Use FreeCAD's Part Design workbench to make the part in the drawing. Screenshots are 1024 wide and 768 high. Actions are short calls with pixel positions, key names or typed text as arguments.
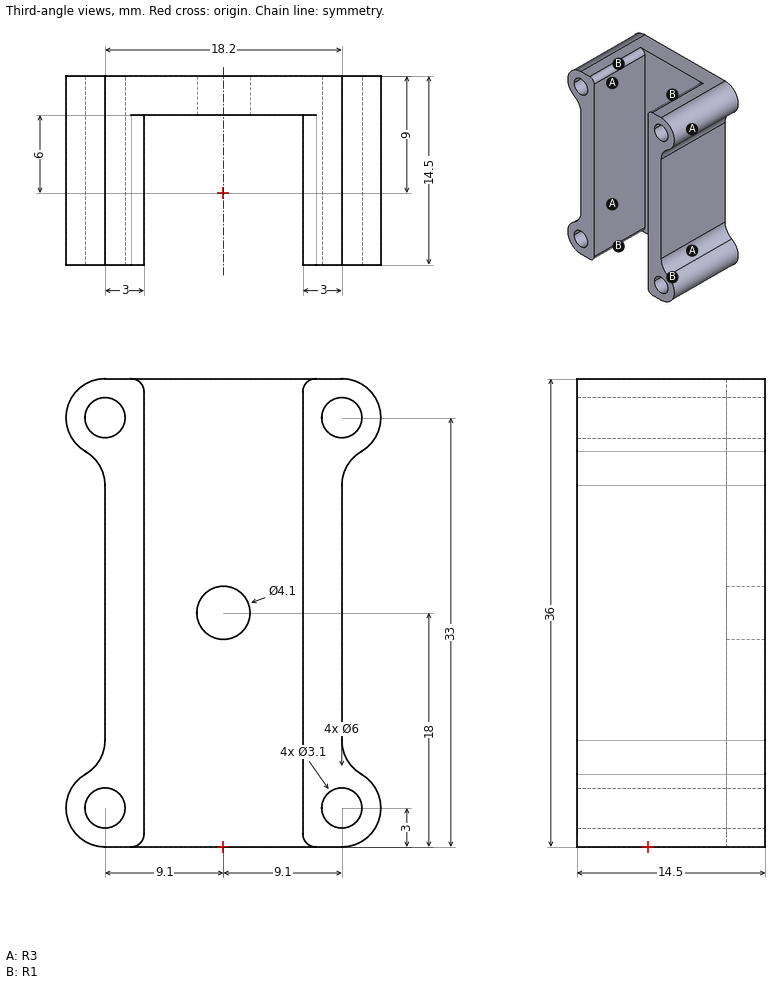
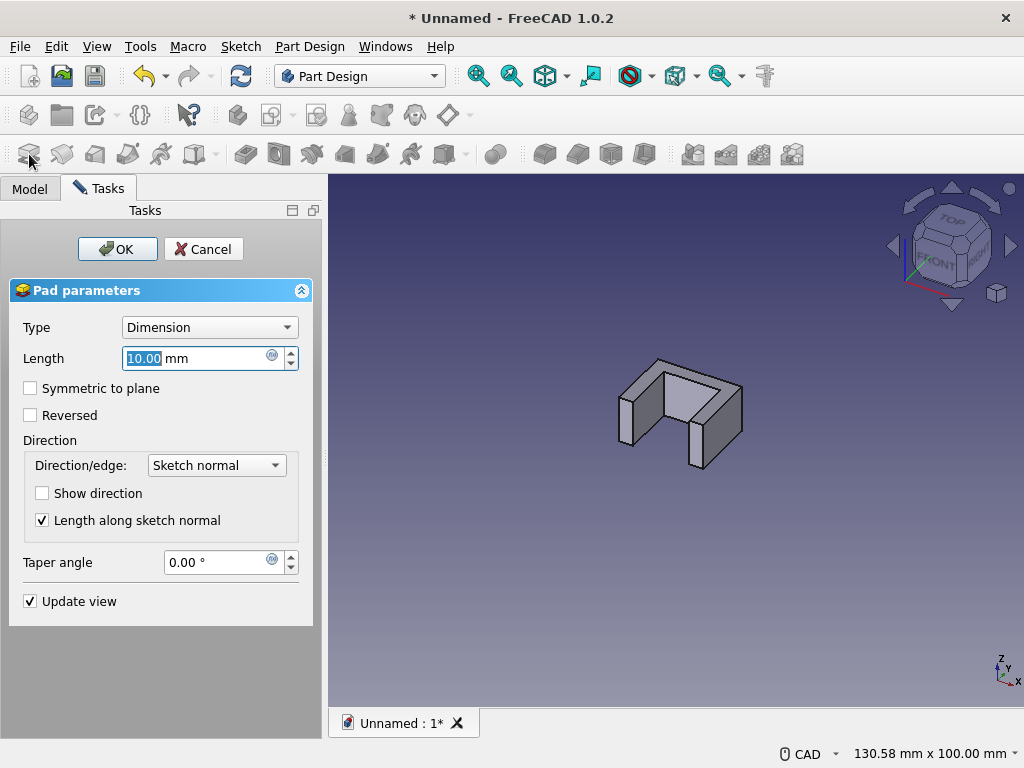
text(36)
key(Tab)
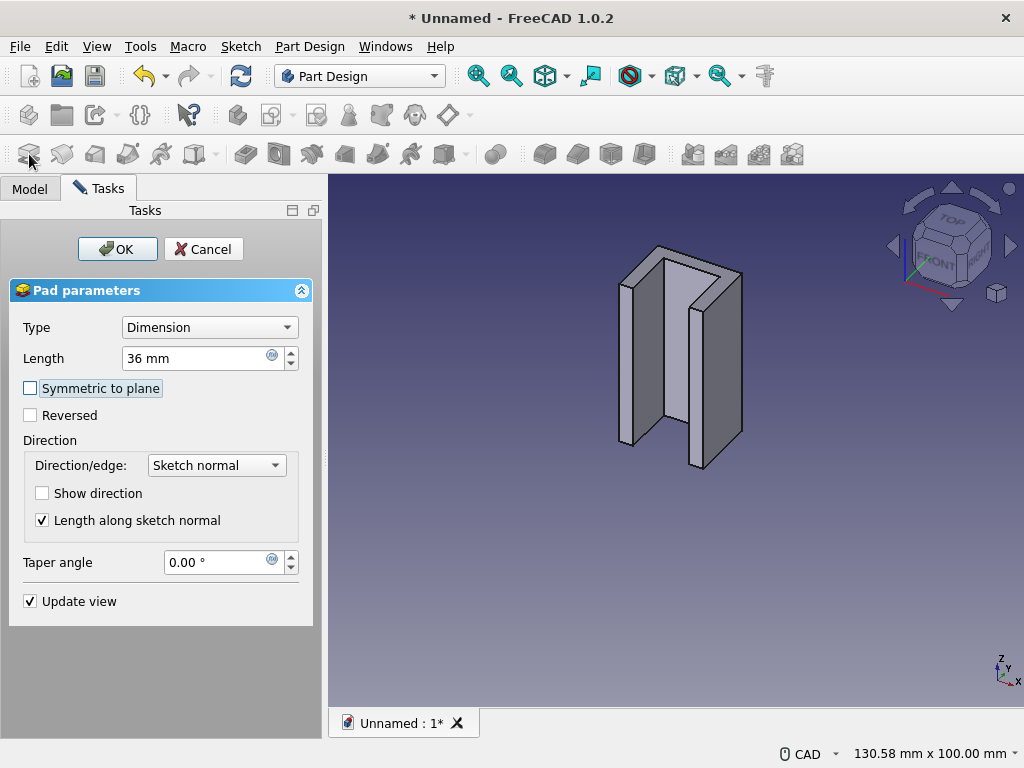
click(118, 249)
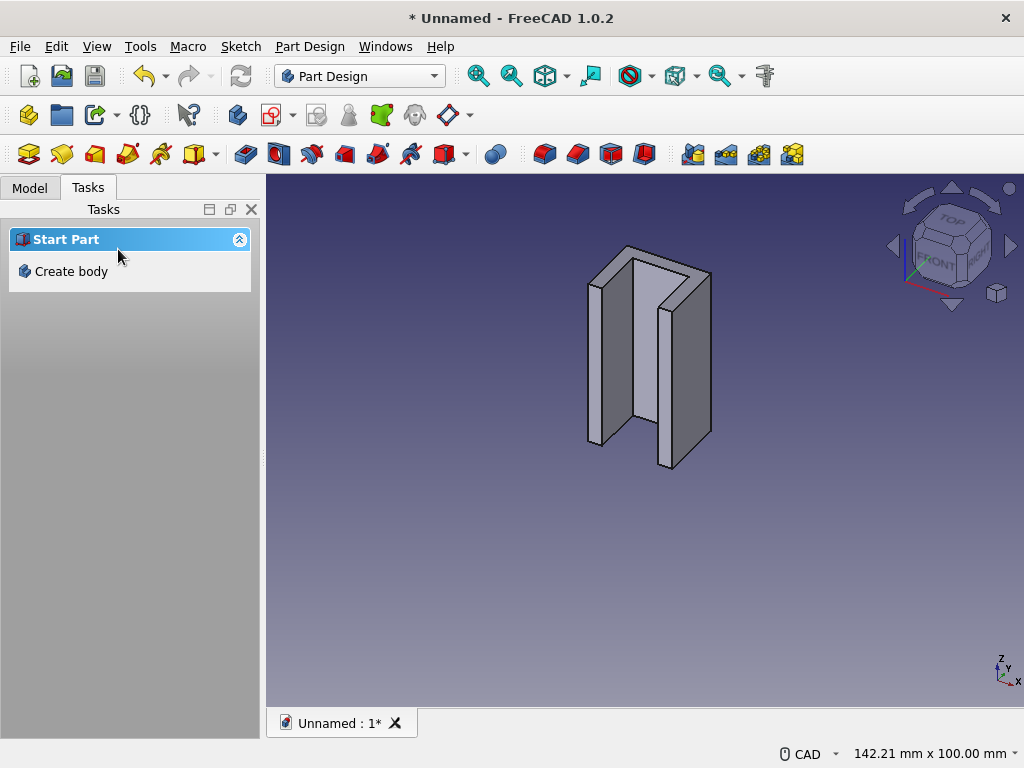
click(479, 76)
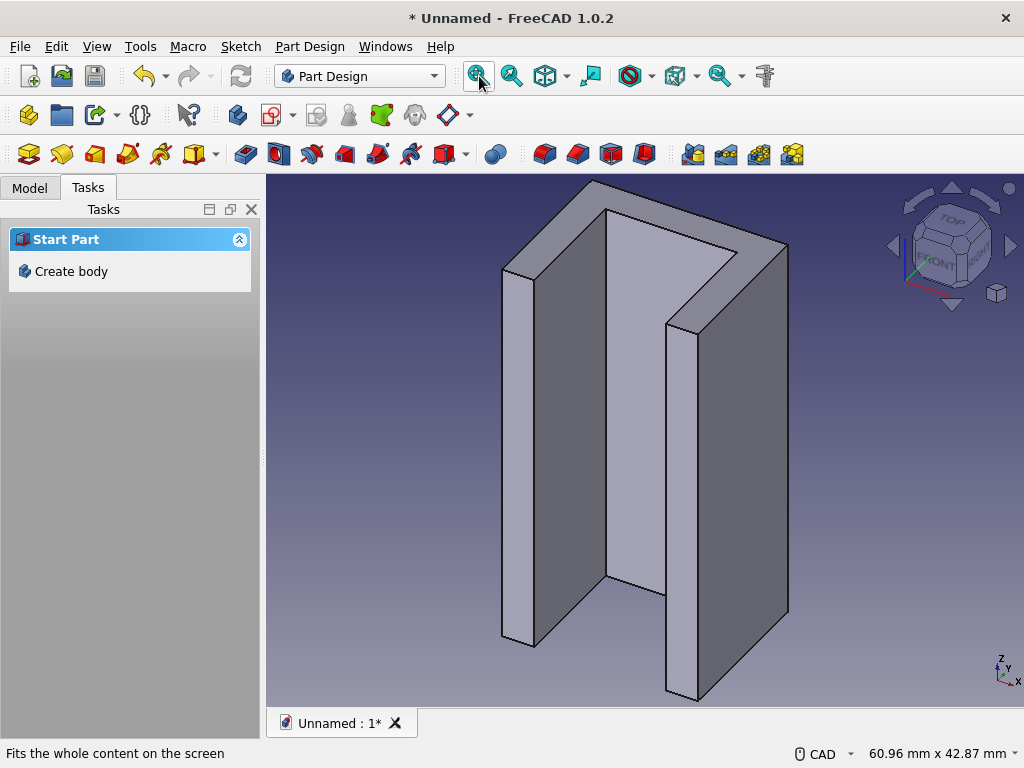
key(4)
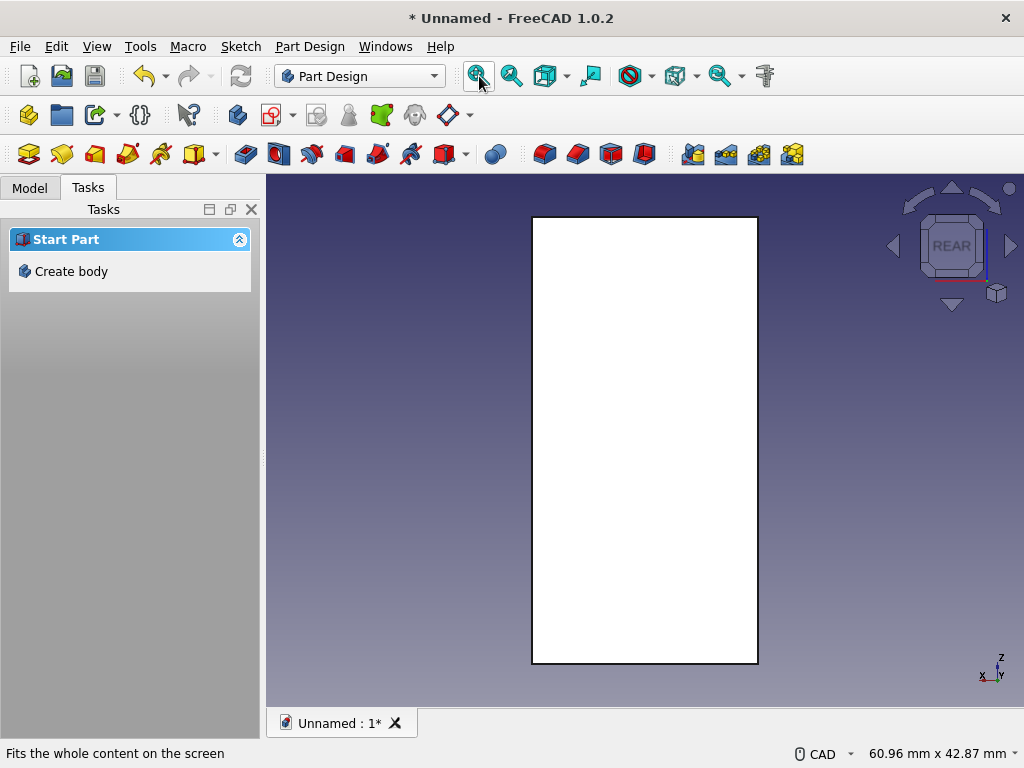
click(645, 376)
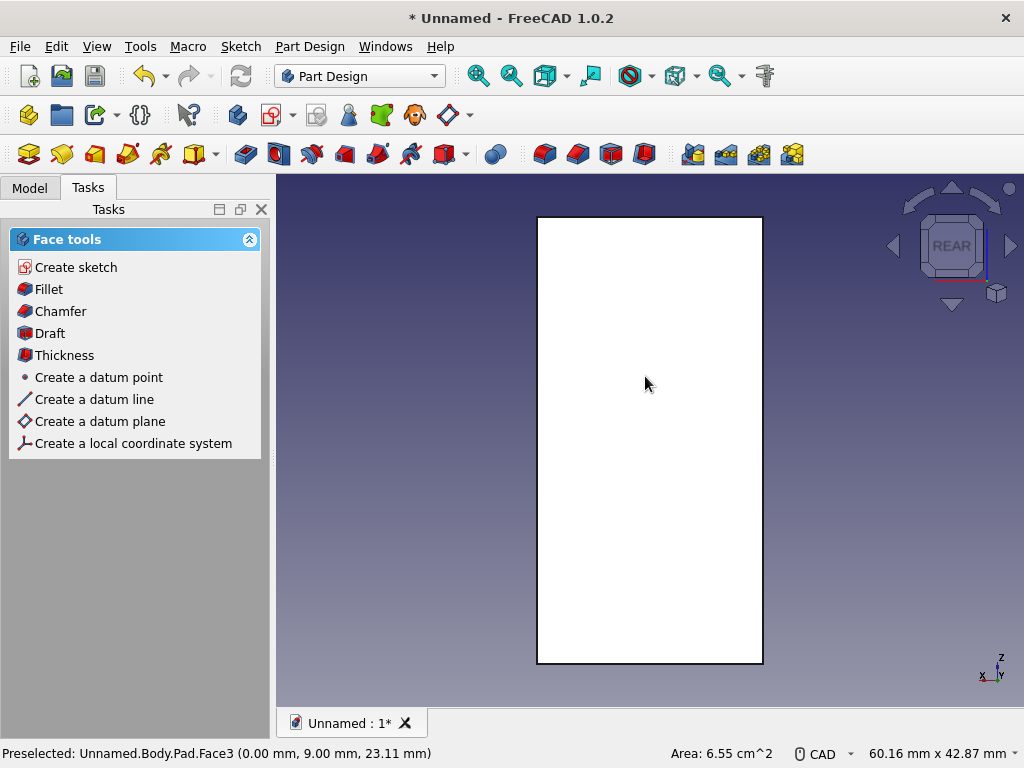
click(270, 116)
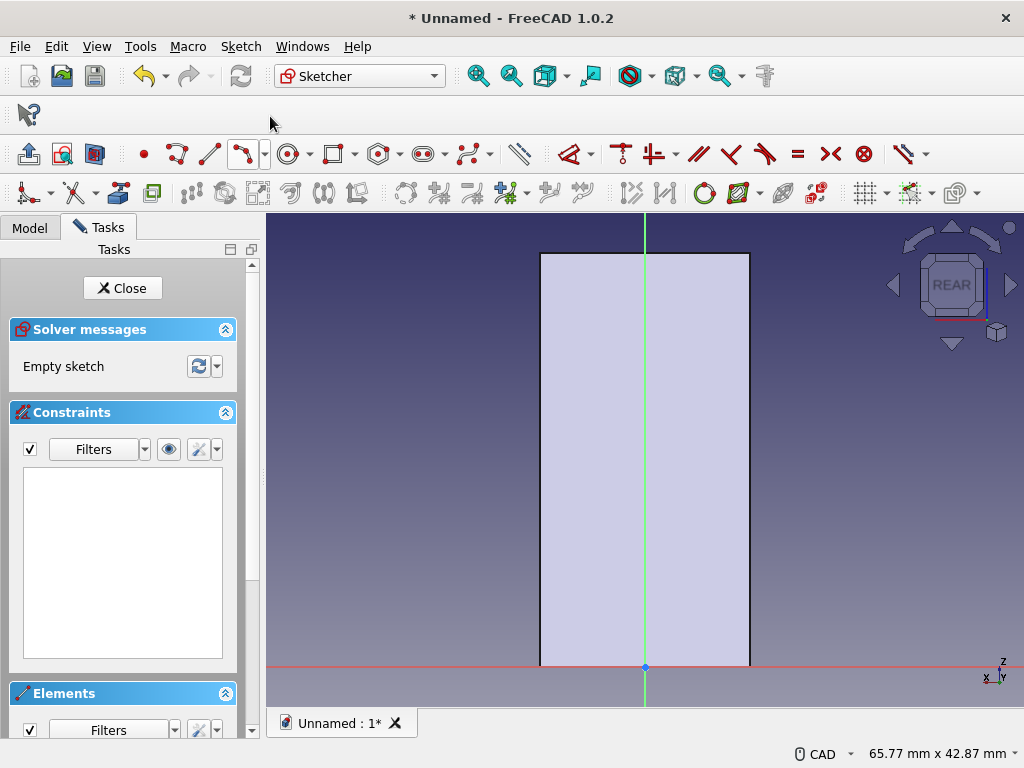
scroll(294, 460, down, 1)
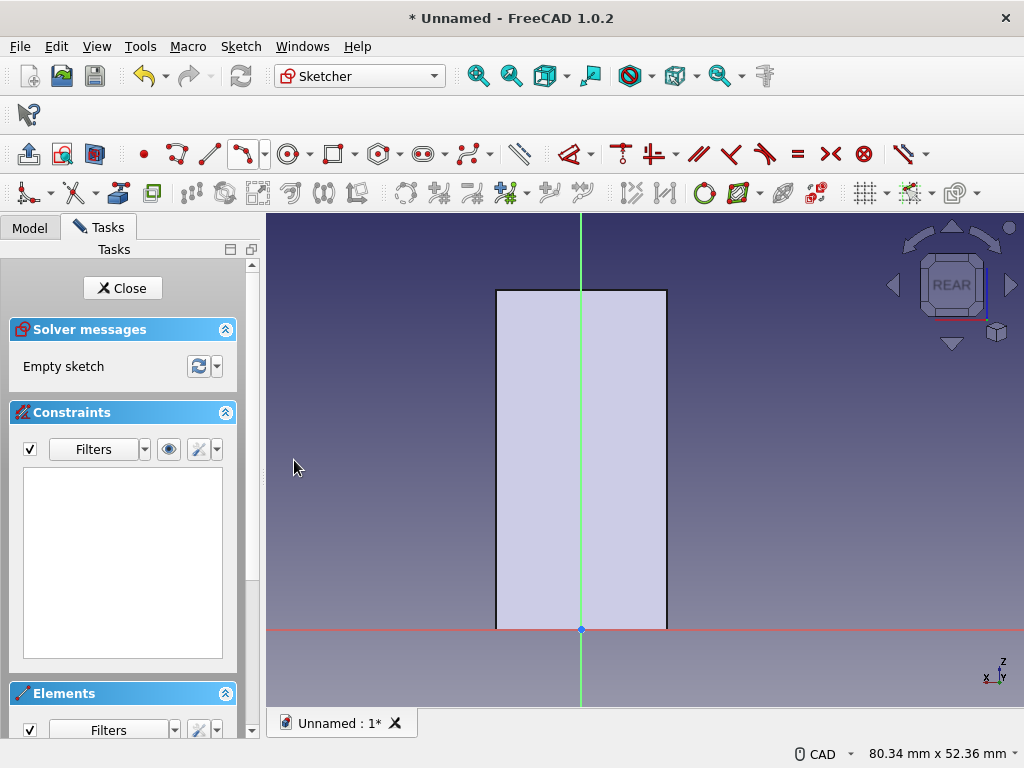
click(288, 154)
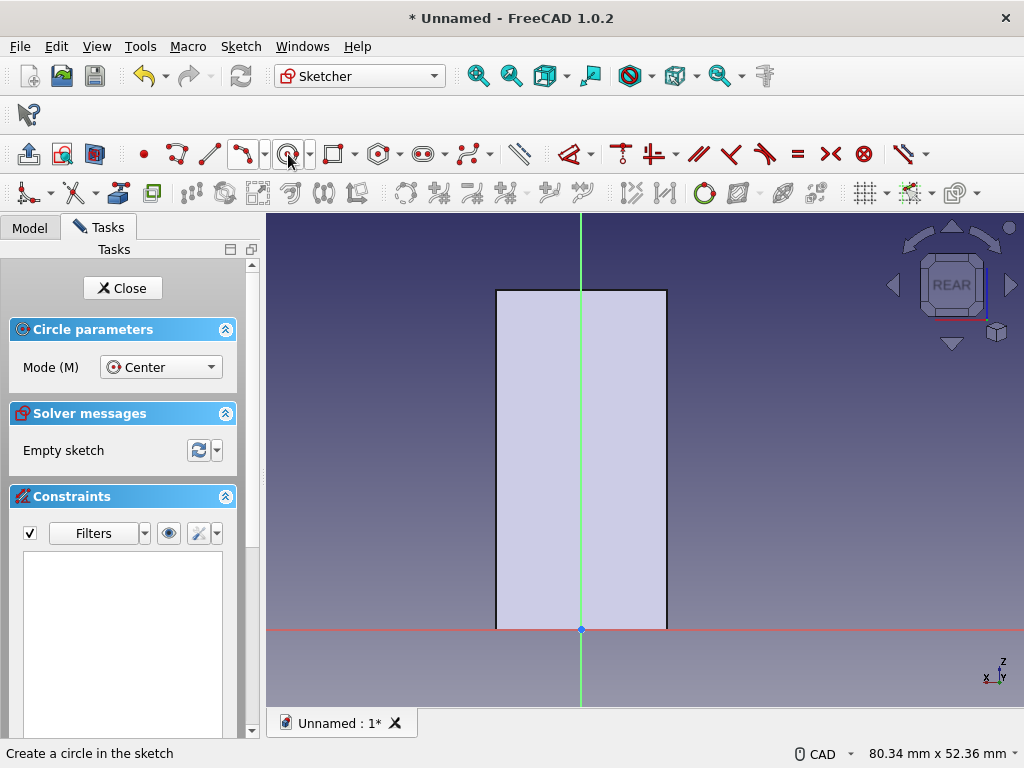
click(496, 602)
click(516, 582)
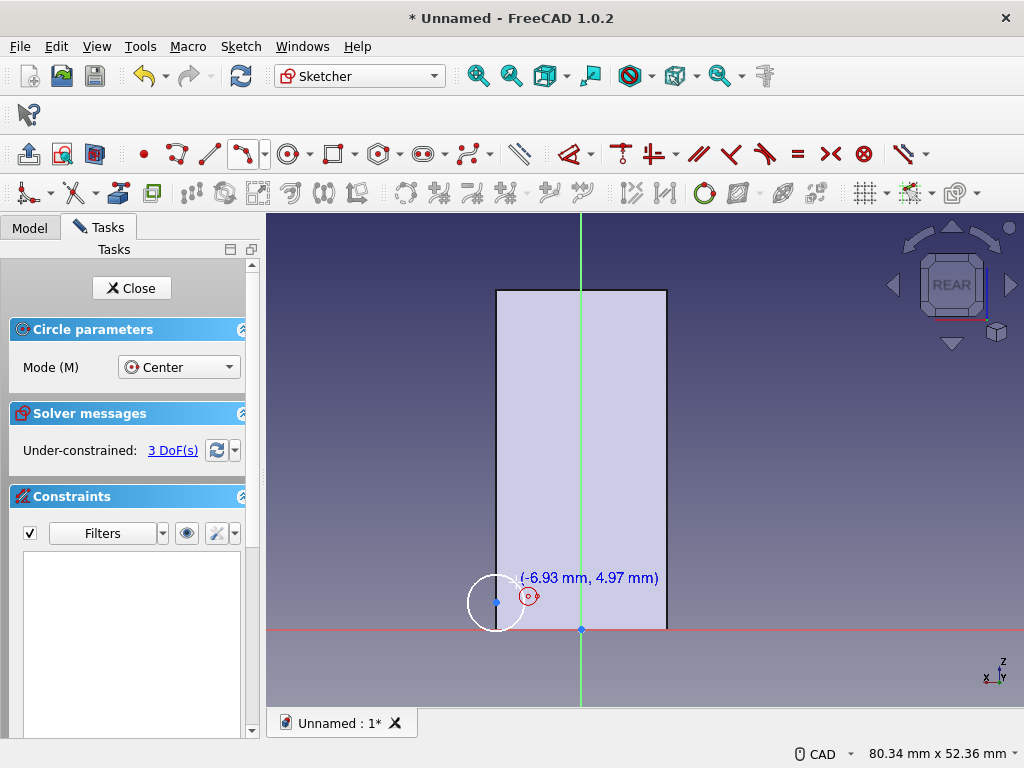
click(667, 602)
click(687, 582)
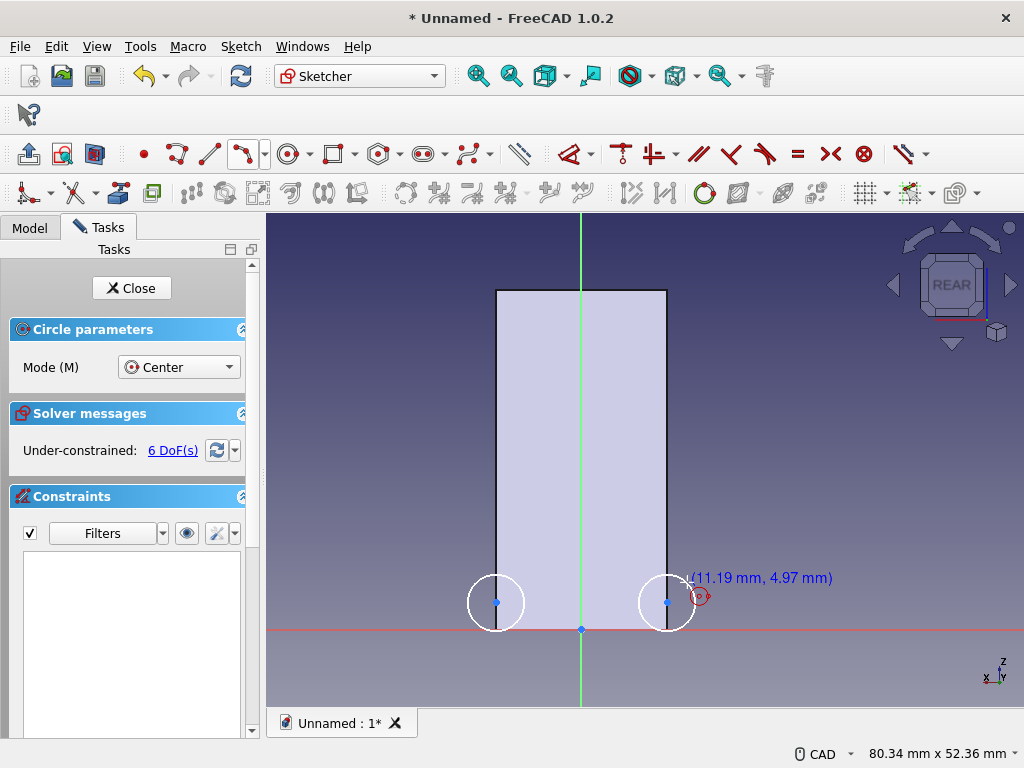
click(496, 319)
click(516, 299)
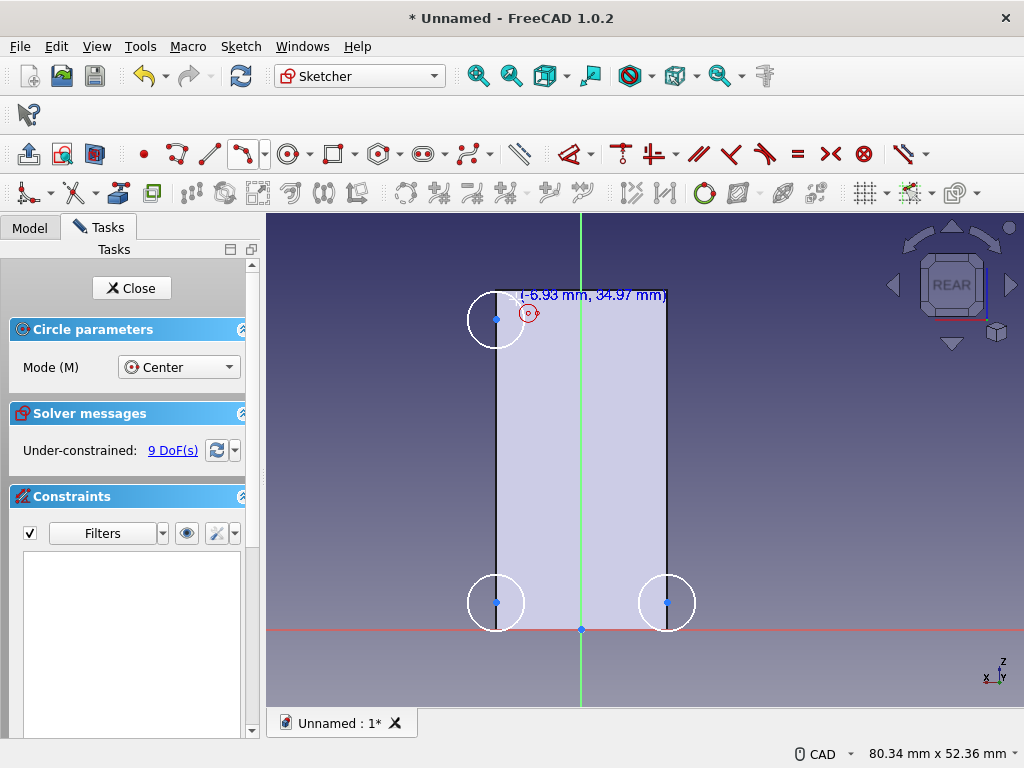
click(667, 319)
click(687, 299)
key(Escape)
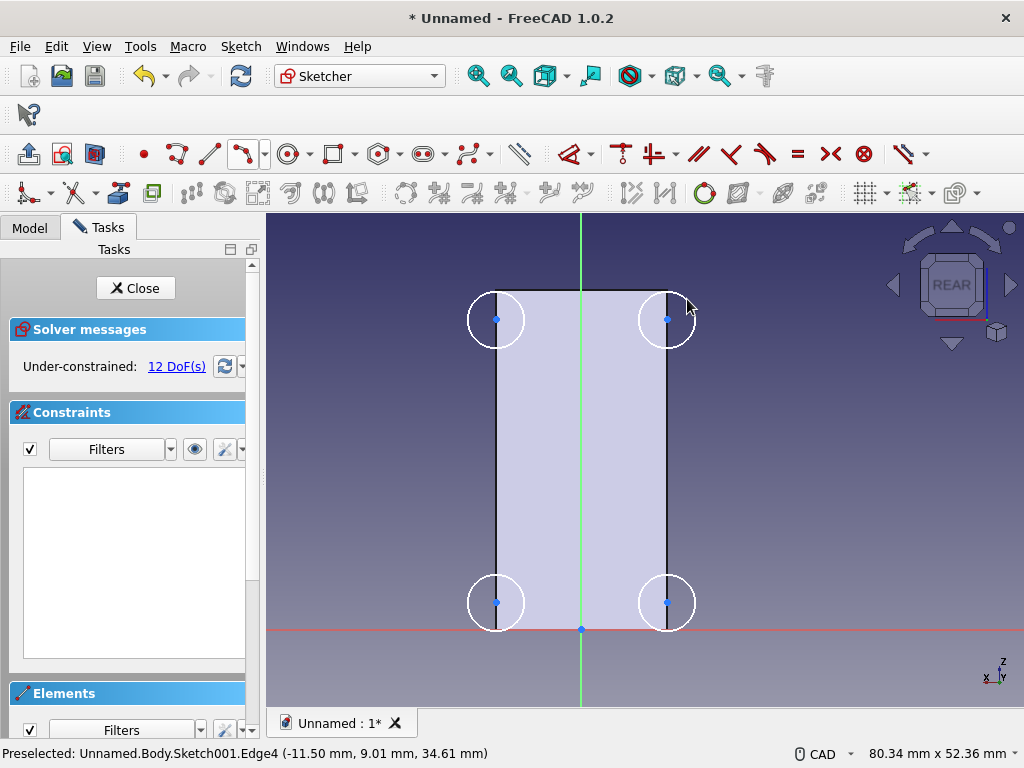
click(516, 583)